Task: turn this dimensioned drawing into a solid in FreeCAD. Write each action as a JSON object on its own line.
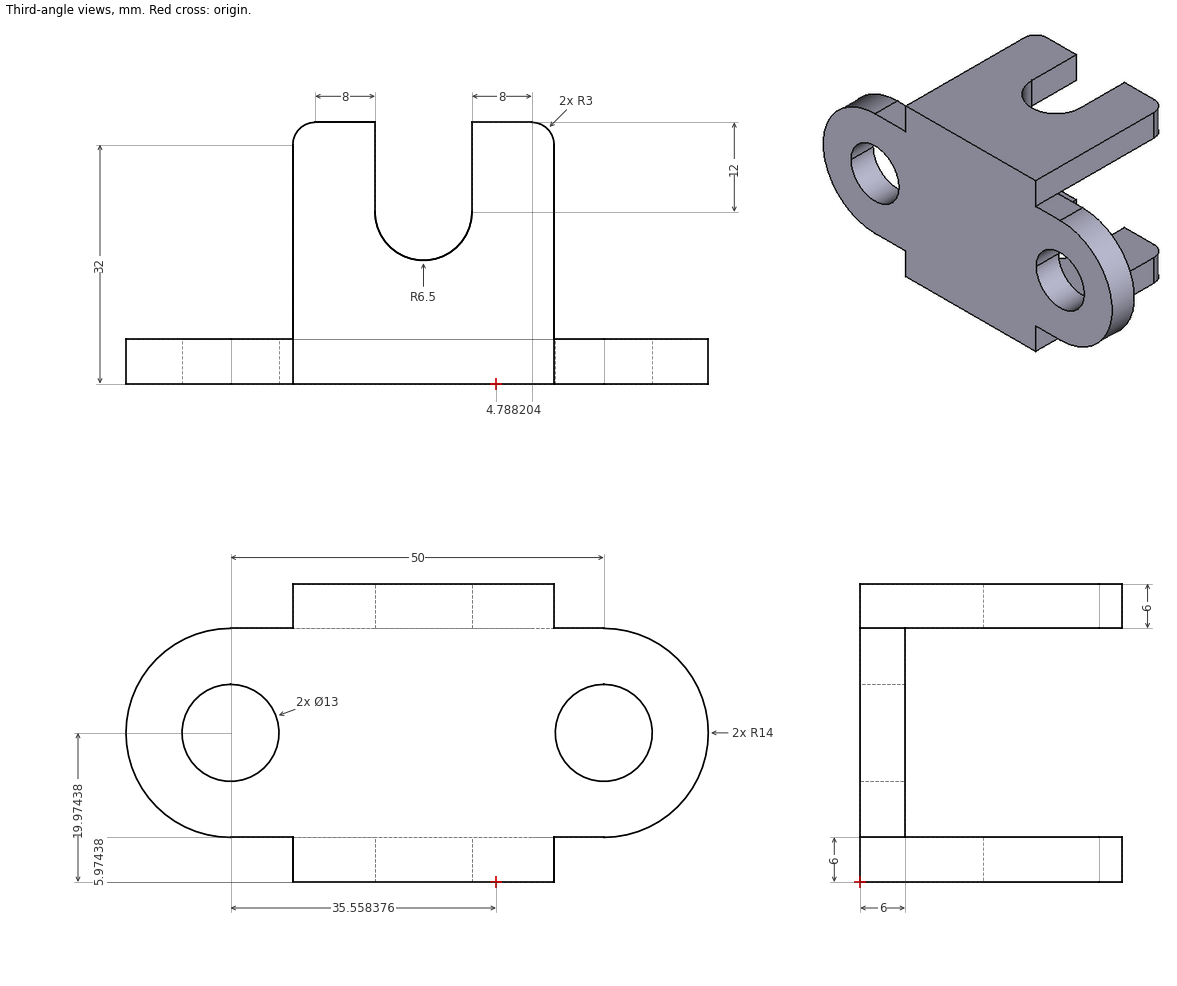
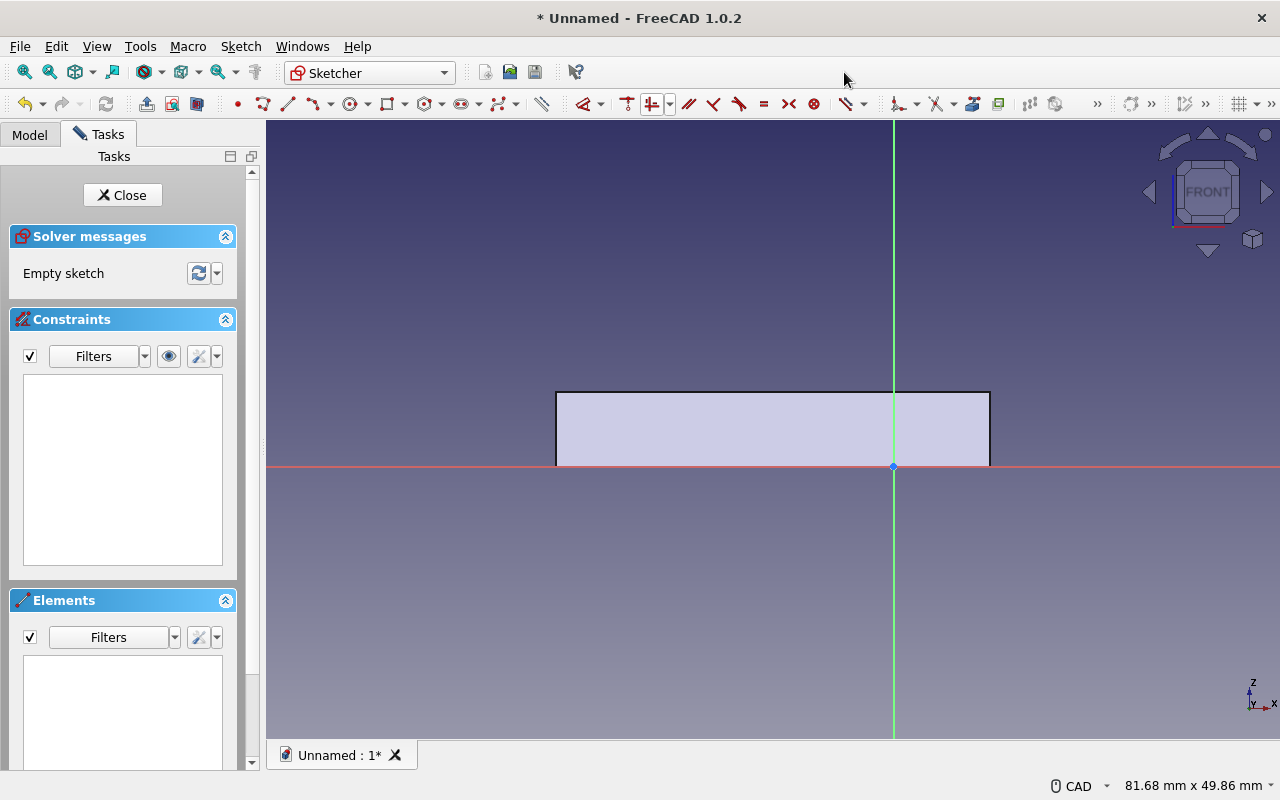
{"action": "scroll", "coordinate": [634, 641], "scroll_direction": "down", "scroll_amount": 3}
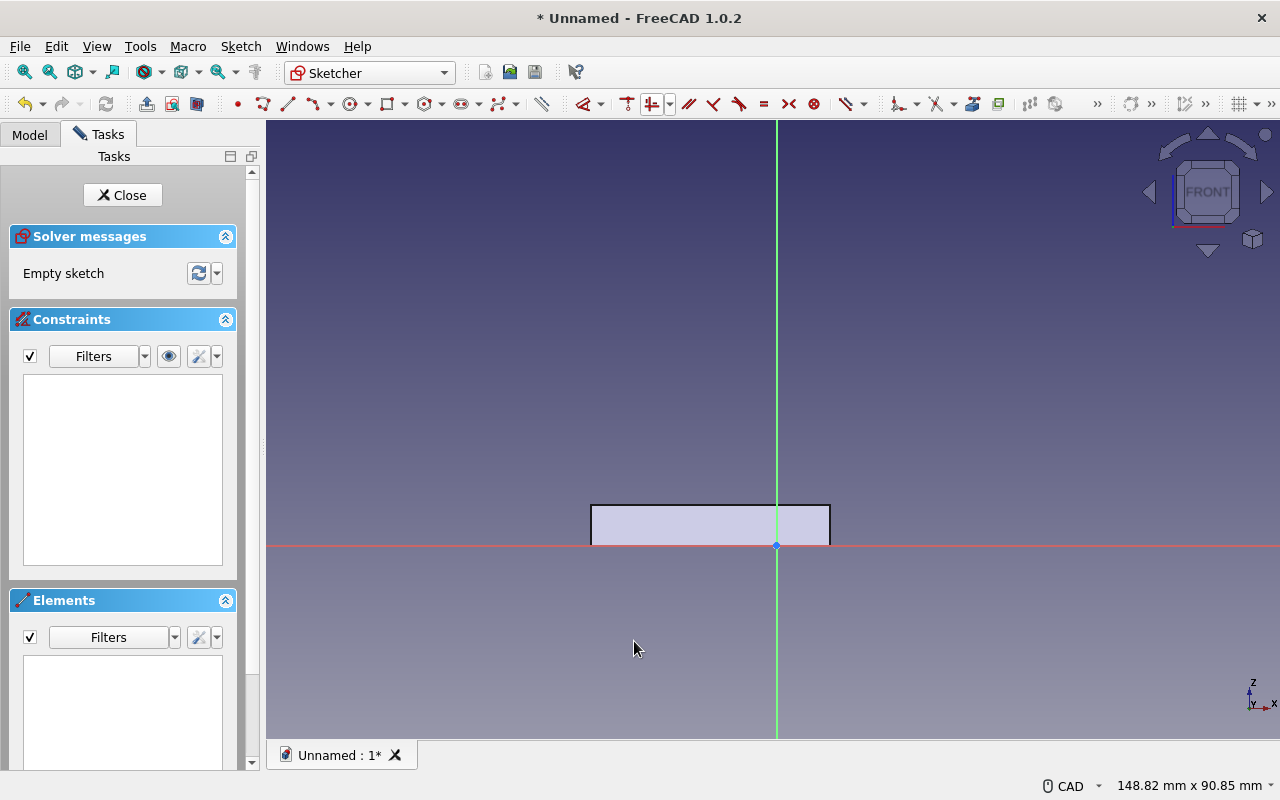
{"action": "left_click", "coordinate": [460, 104]}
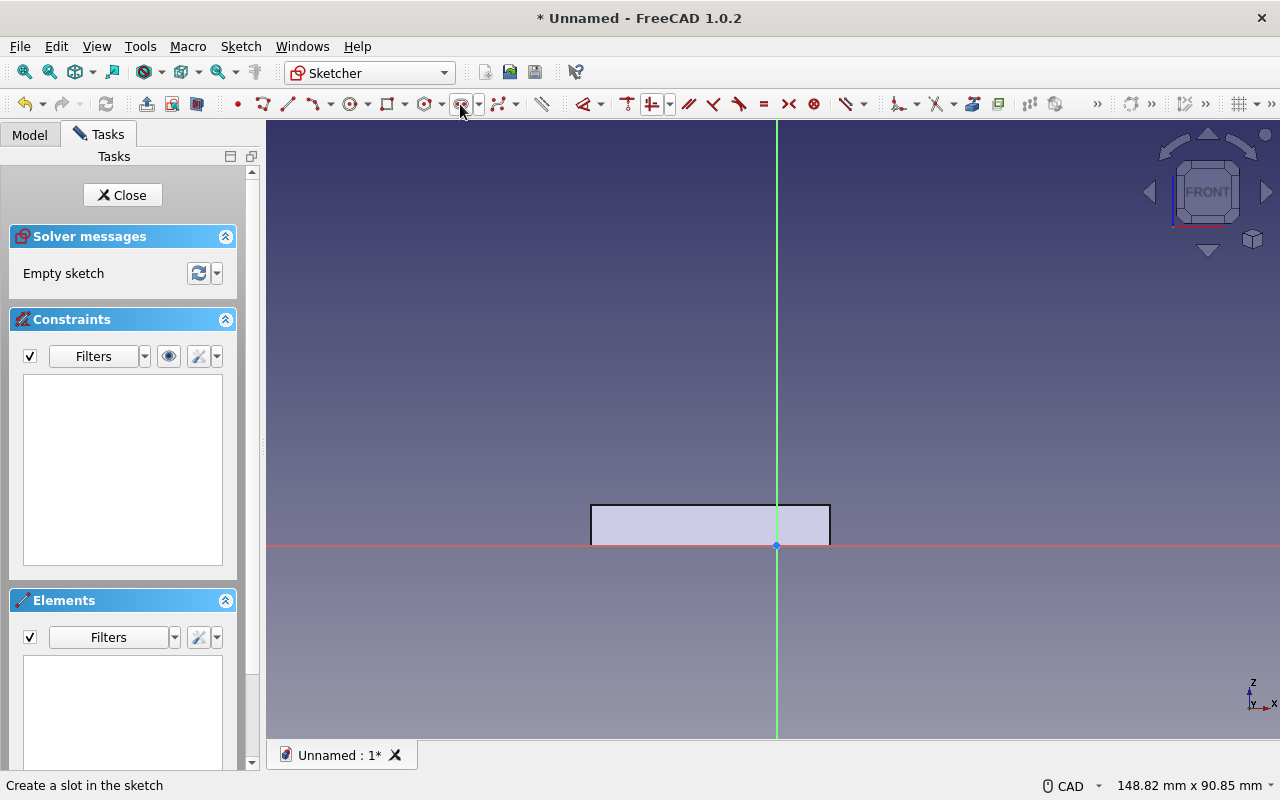
{"action": "left_click", "coordinate": [534, 410]}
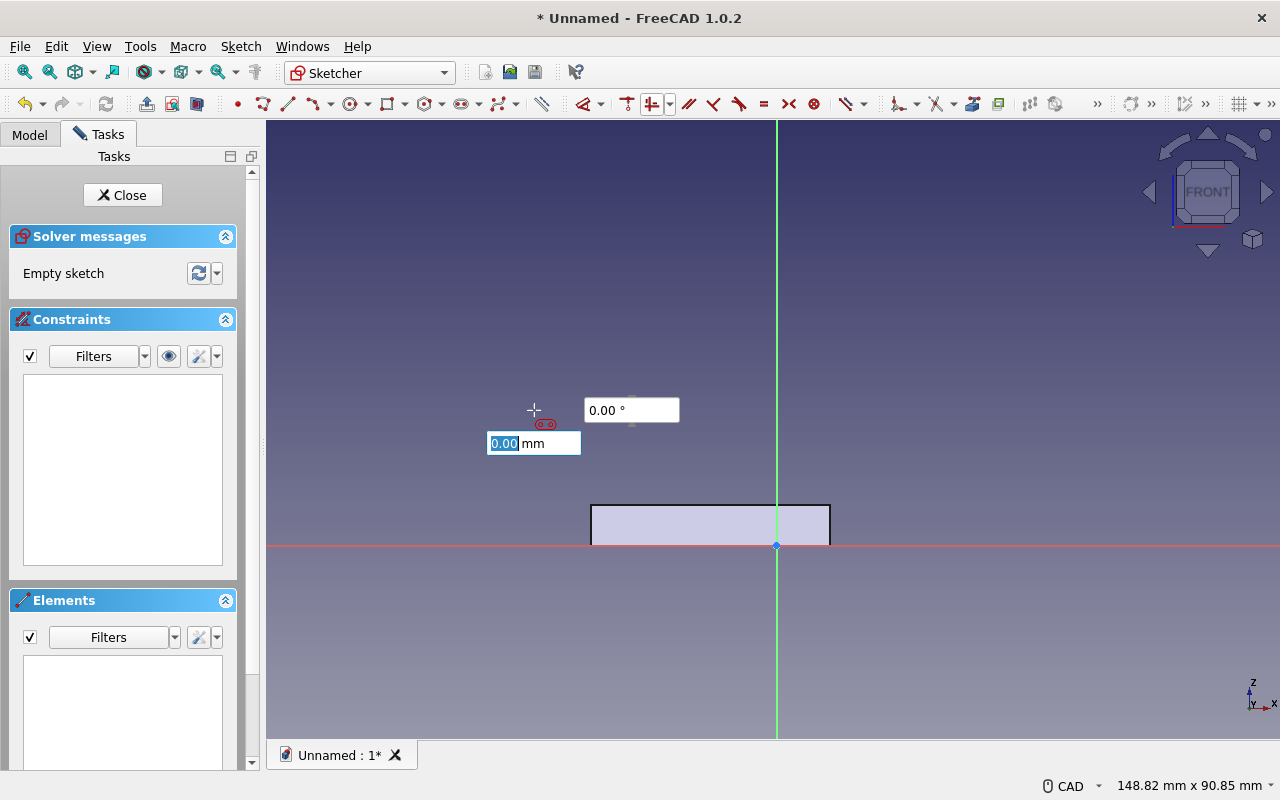
{"action": "left_click", "coordinate": [875, 410]}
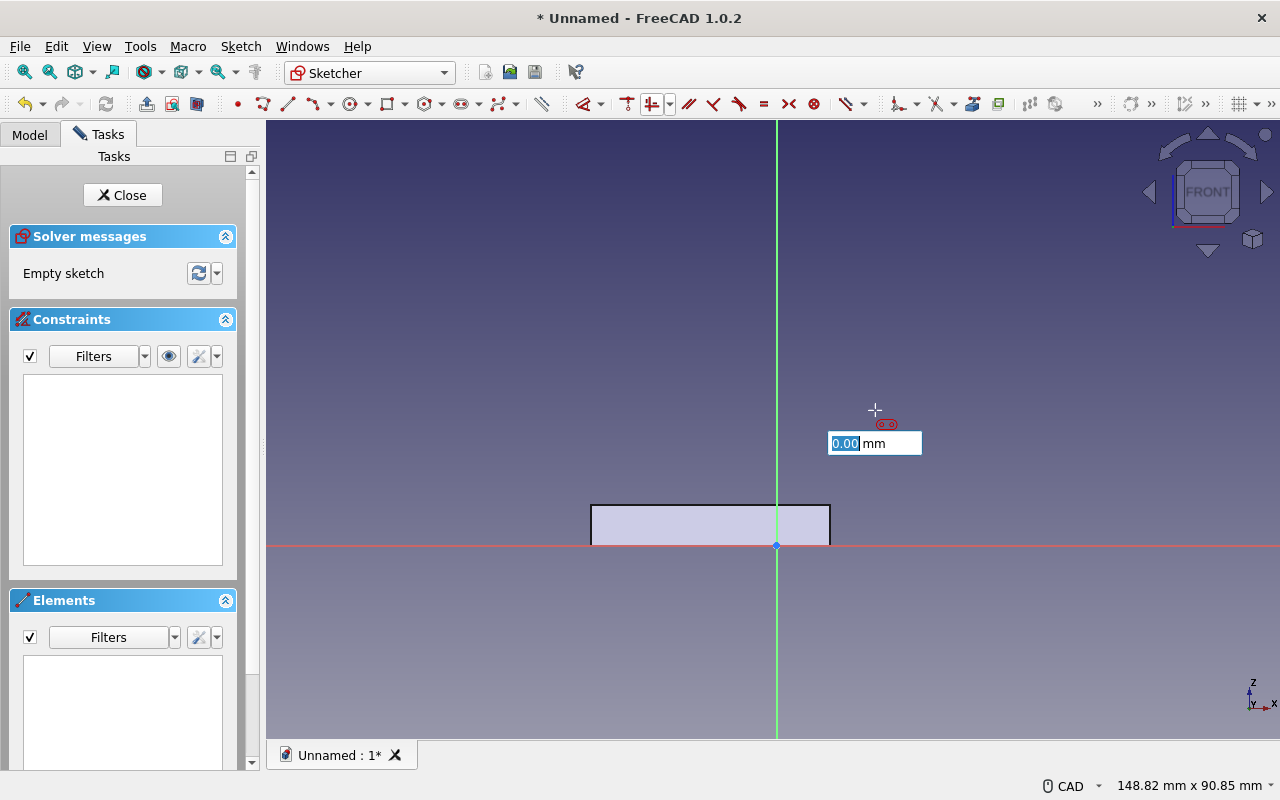
{"action": "left_click", "coordinate": [705, 505]}
{"action": "key", "text": "Escape"}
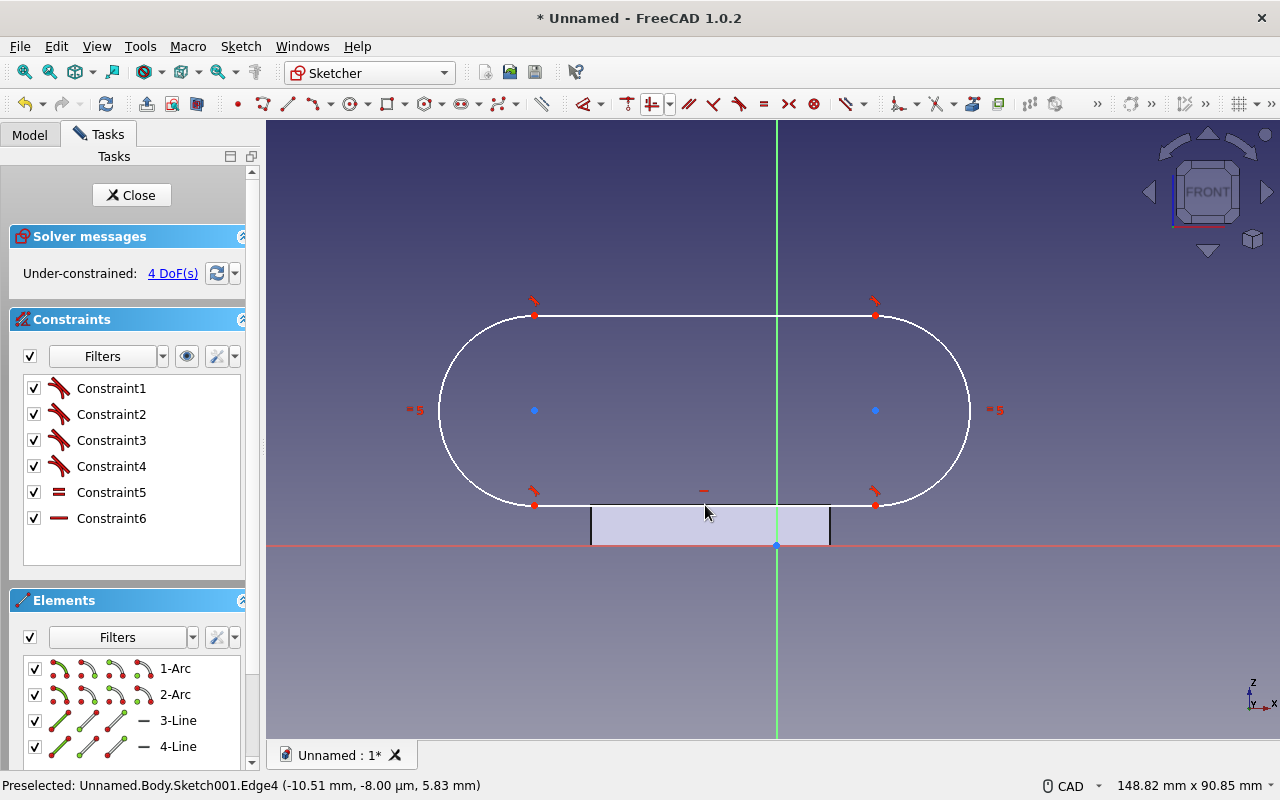
{"action": "left_click", "coordinate": [582, 104]}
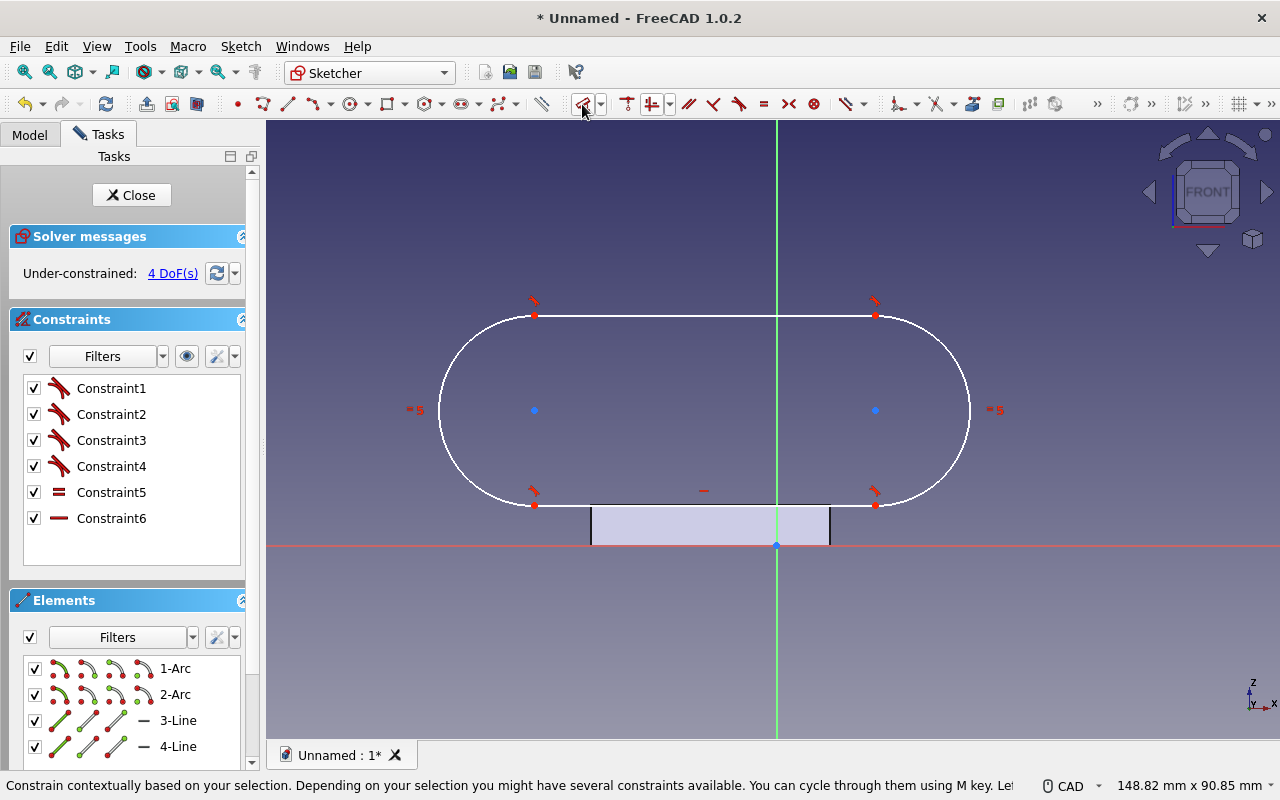
{"action": "left_click", "coordinate": [457, 355]}
{"action": "left_click", "coordinate": [431, 336]}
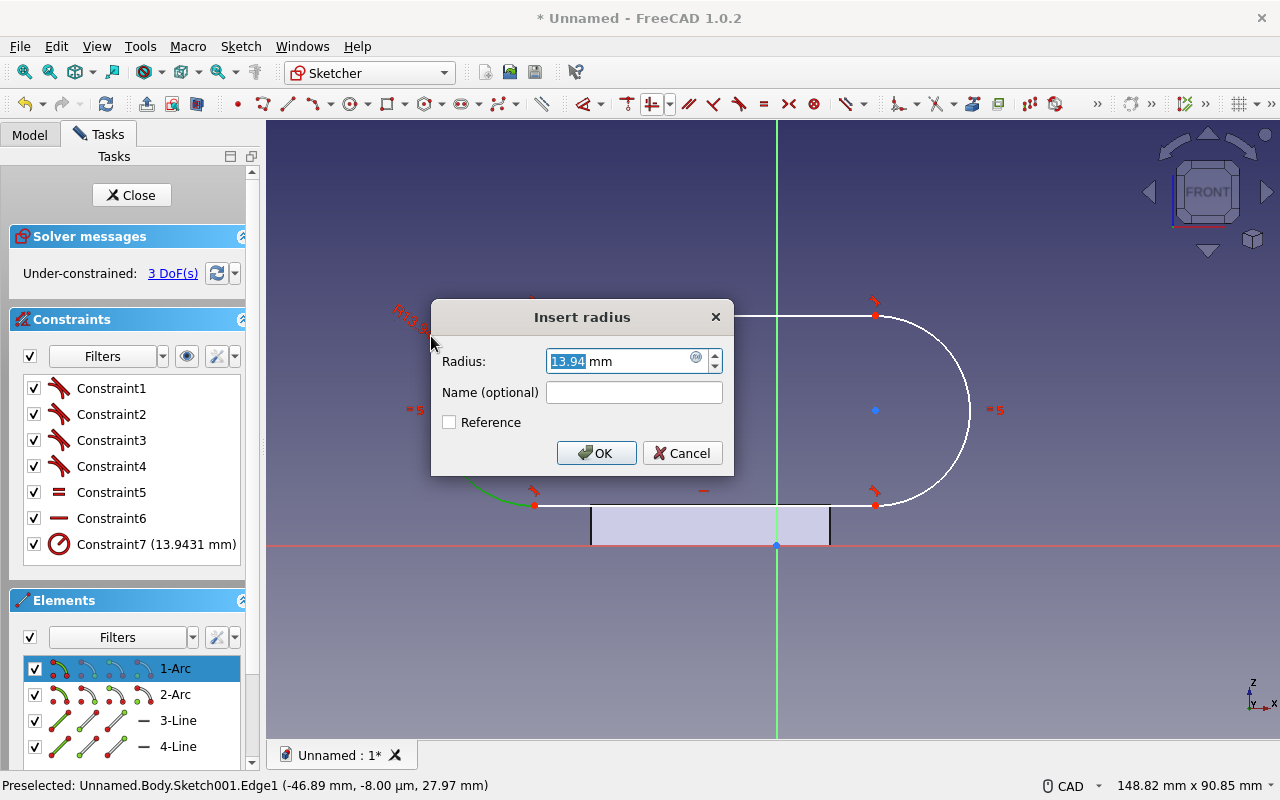
{"action": "type", "text": "14"}
{"action": "key", "text": "Return"}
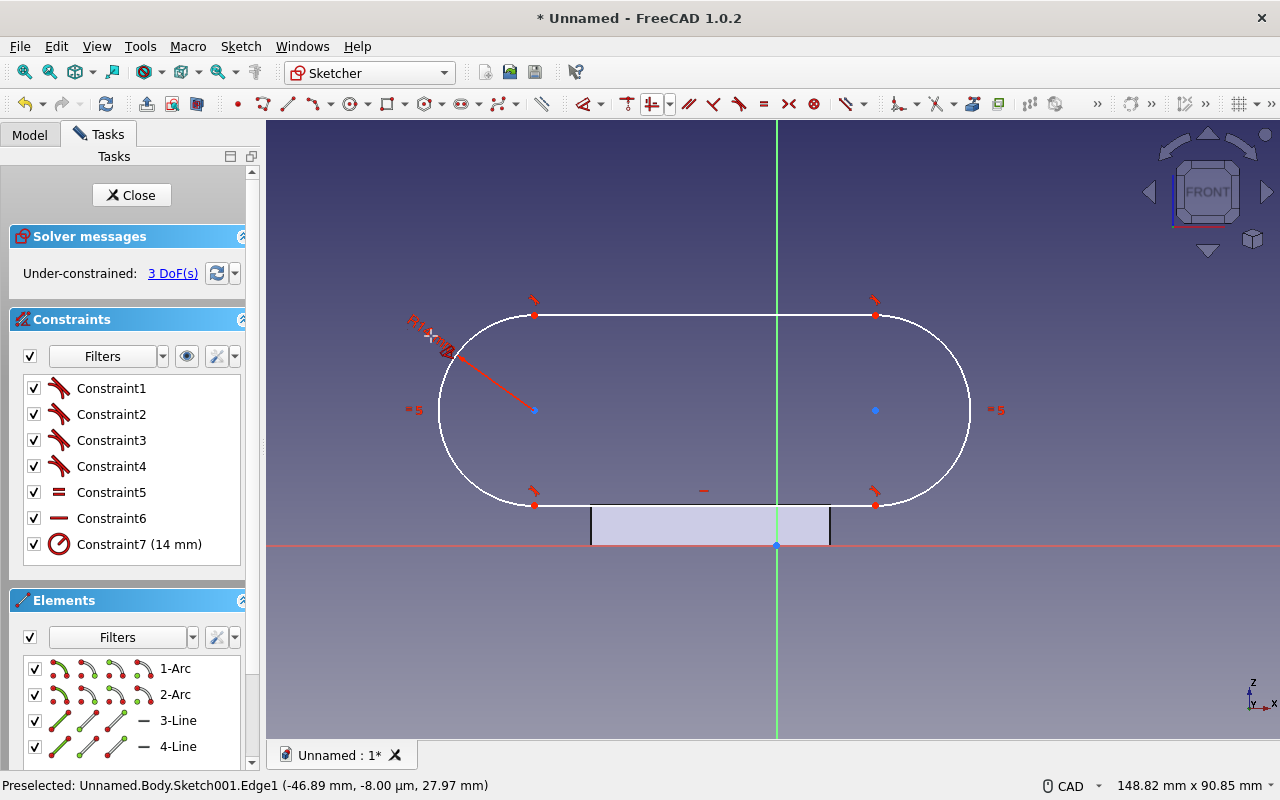
{"action": "left_click", "coordinate": [636, 315]}
{"action": "left_click", "coordinate": [705, 281]}